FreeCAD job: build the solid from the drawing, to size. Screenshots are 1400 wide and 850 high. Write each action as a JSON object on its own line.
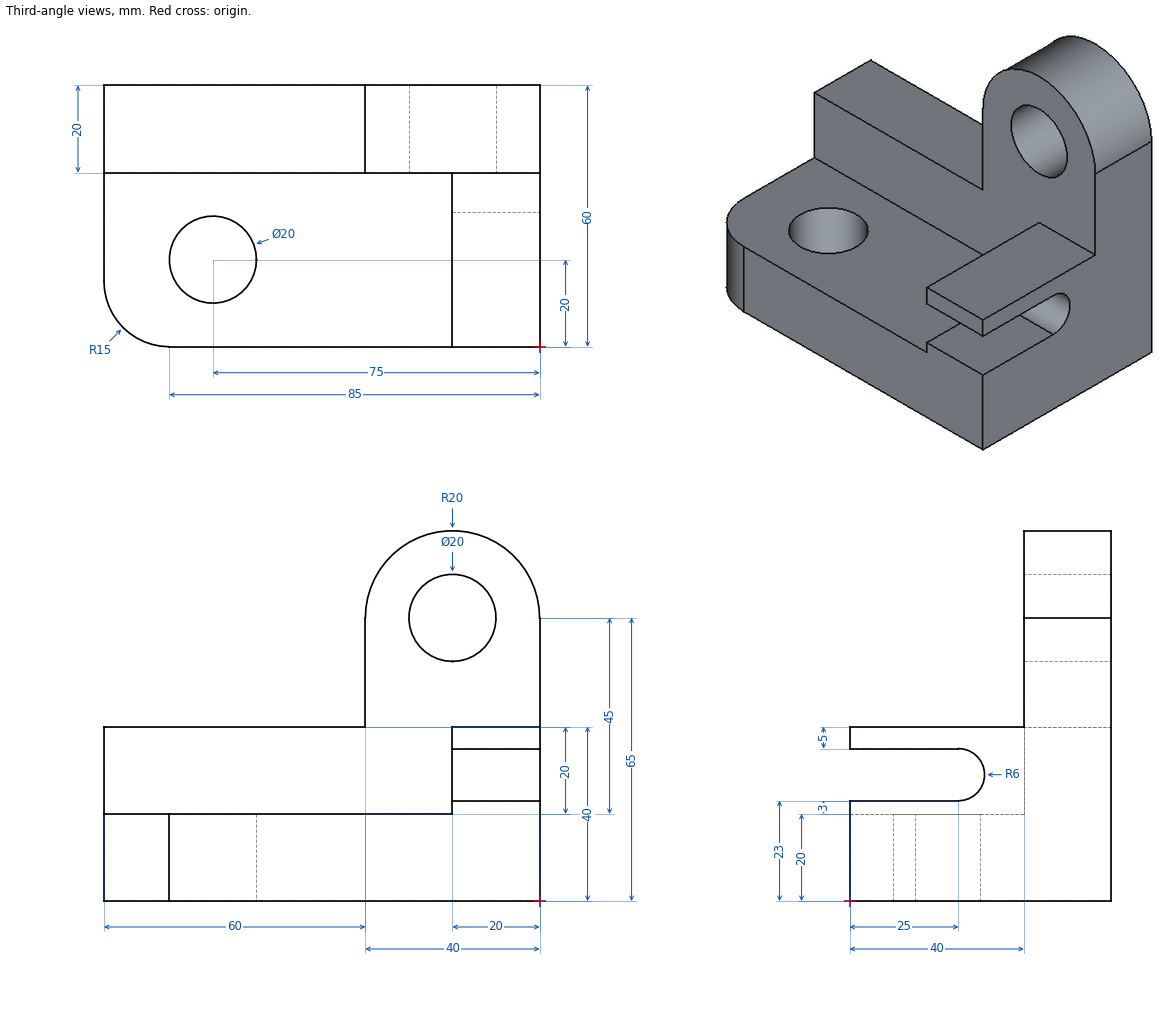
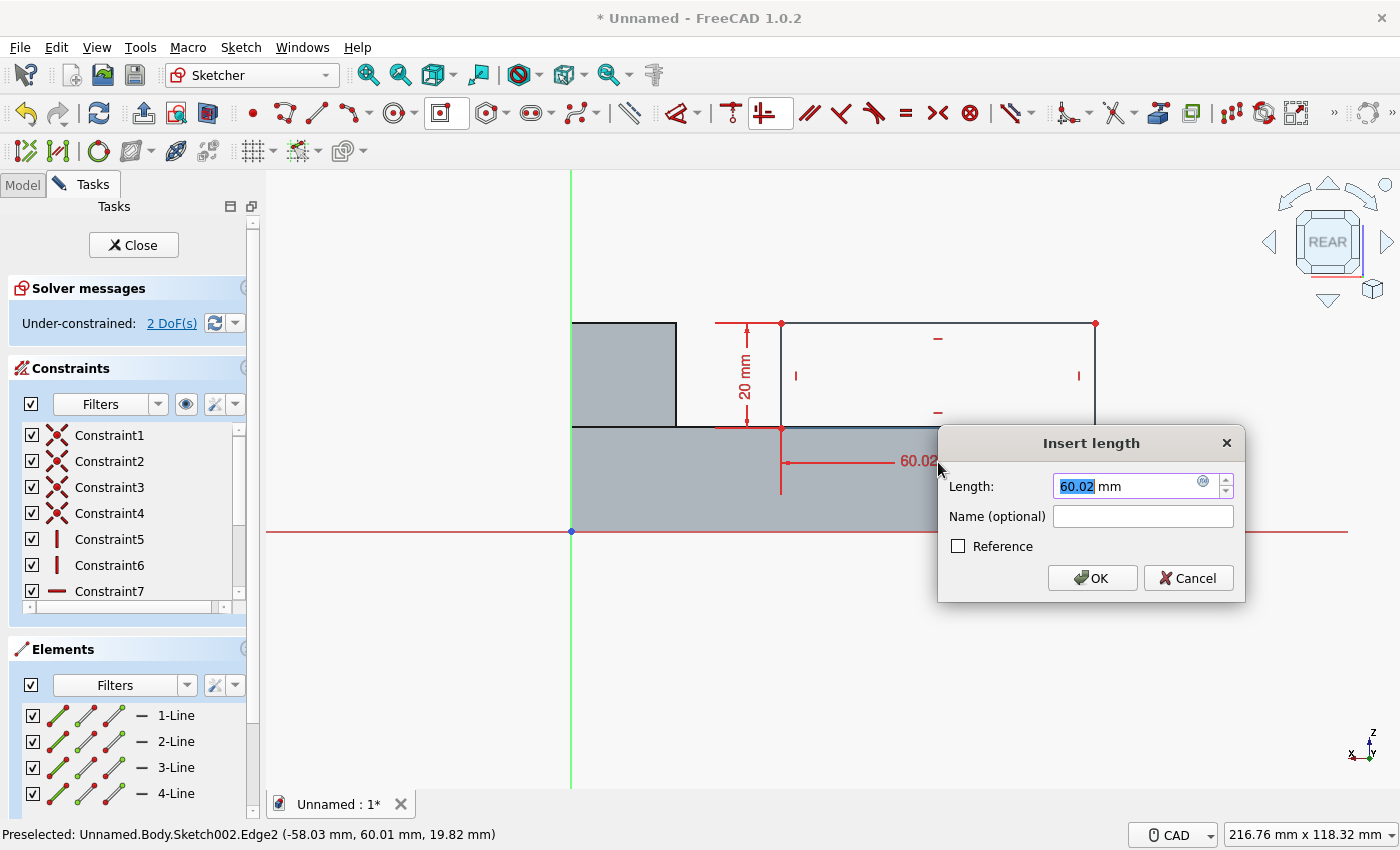
{"action": "type", "text": "60"}
{"action": "key", "text": "Return"}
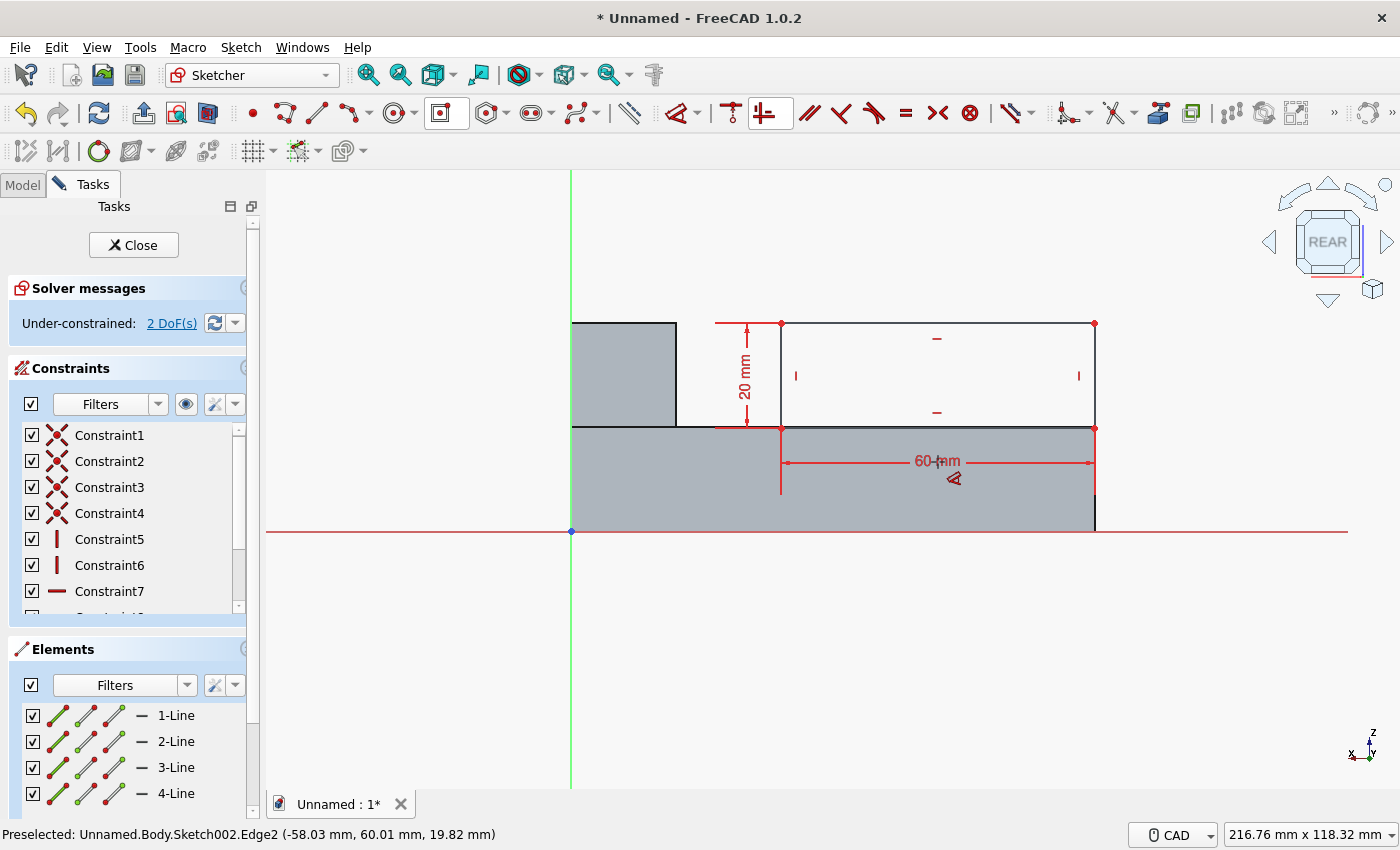
{"action": "left_click", "coordinate": [781, 323]}
{"action": "left_click", "coordinate": [676, 566]}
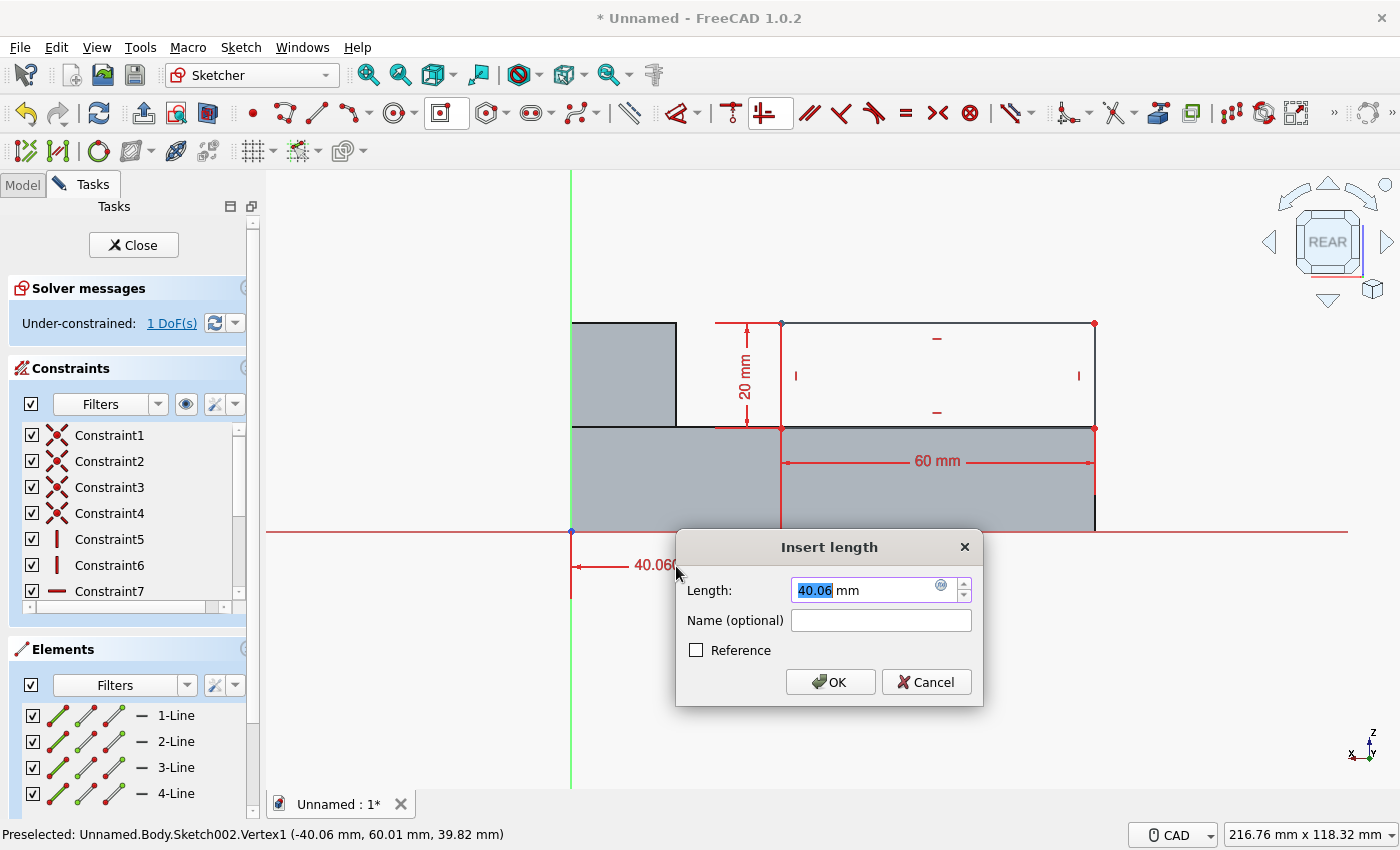
{"action": "type", "text": "40"}
{"action": "key", "text": "Return"}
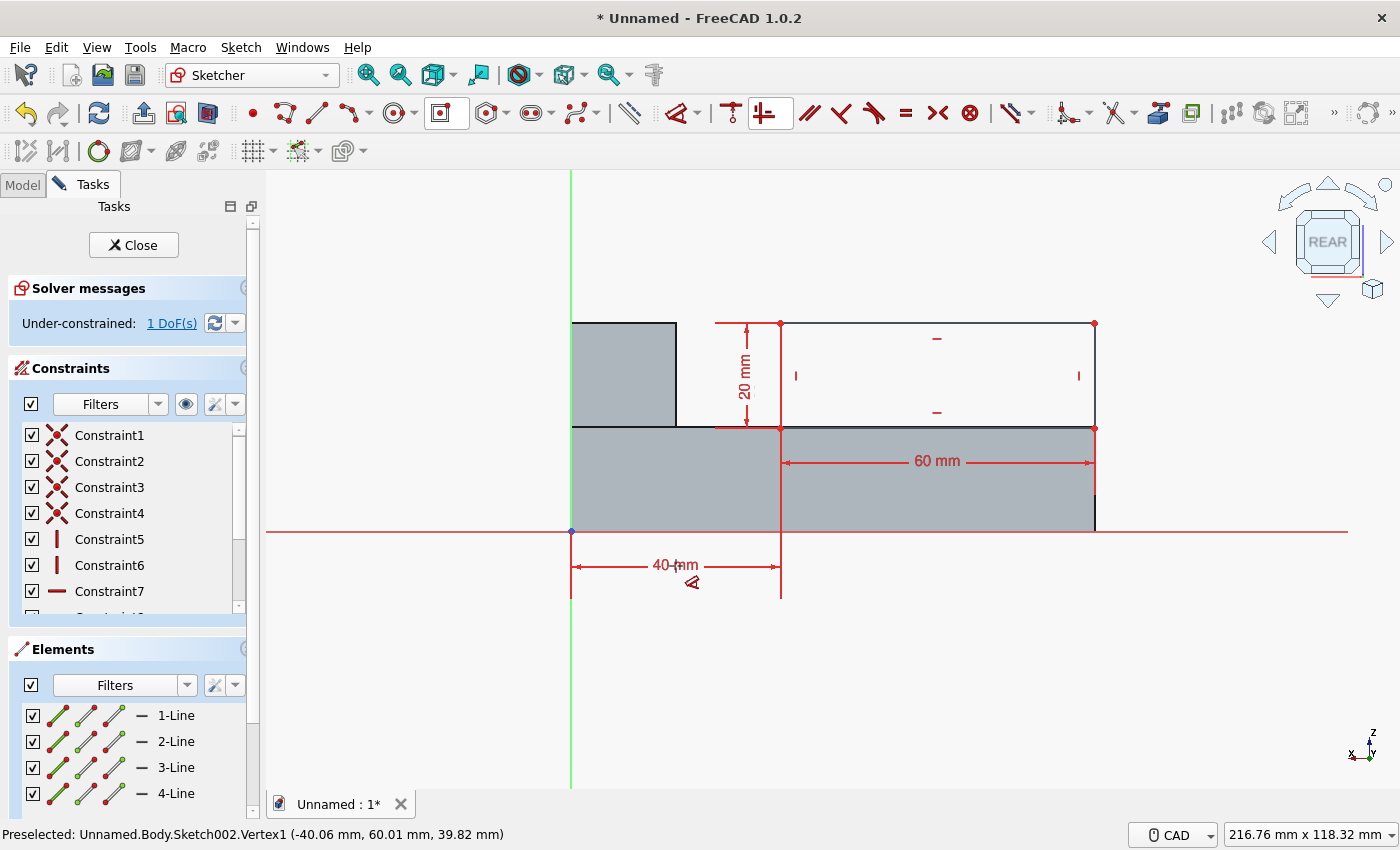
{"action": "left_click", "coordinate": [781, 323]}
{"action": "left_click", "coordinate": [537, 428]}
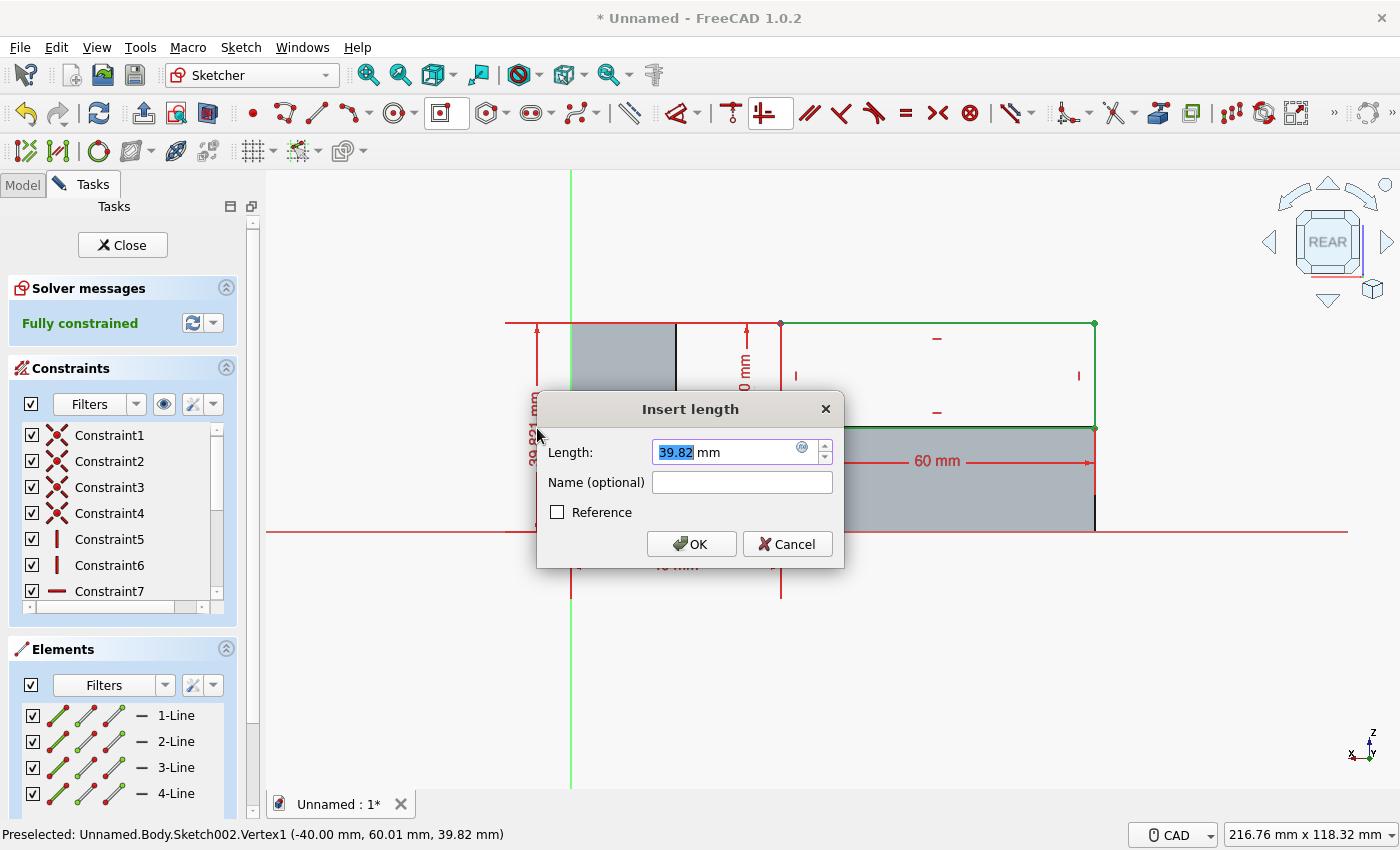
{"action": "type", "text": "40"}
{"action": "key", "text": "Return"}
{"action": "key", "text": "Escape"}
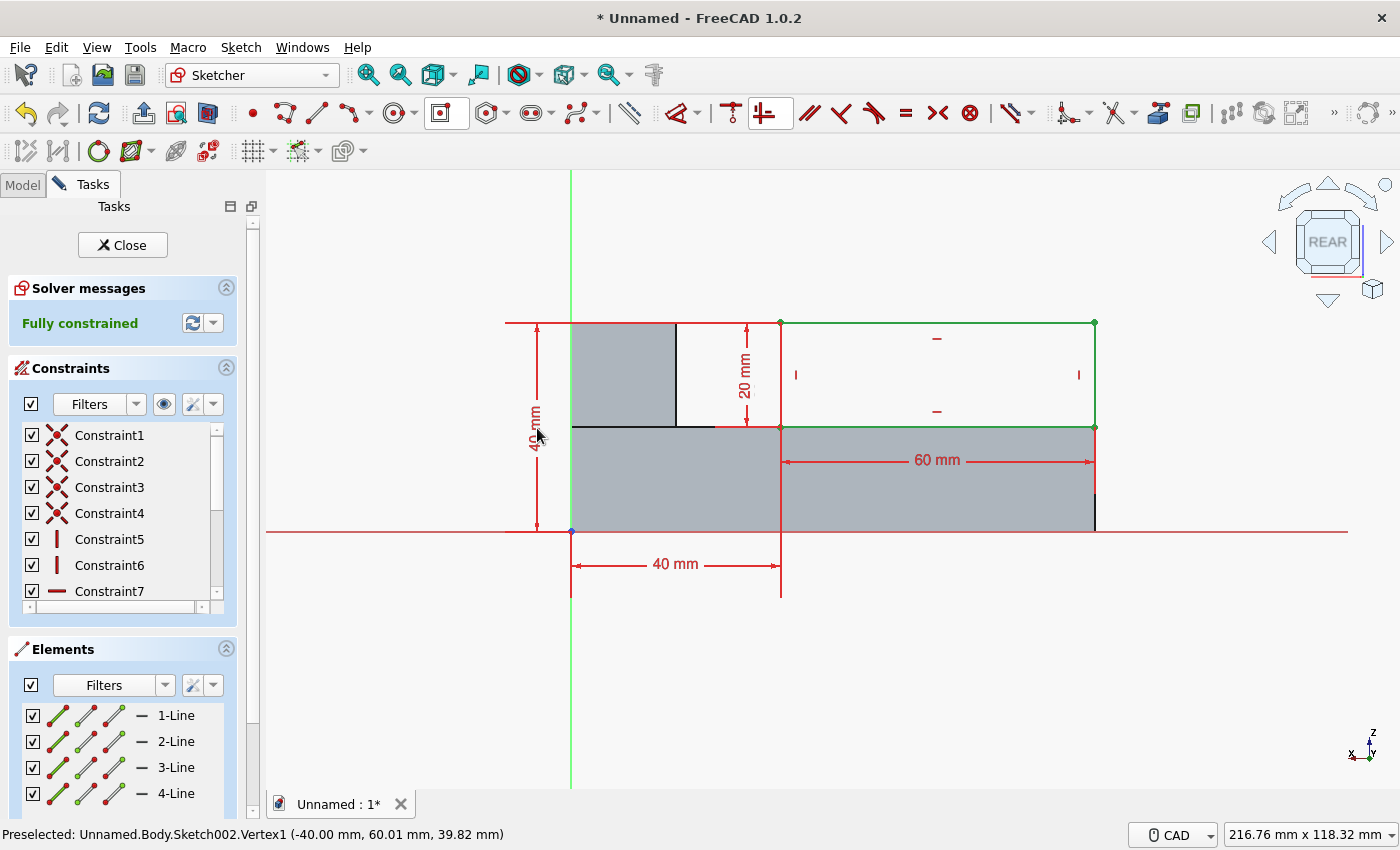
{"action": "left_click", "coordinate": [123, 245]}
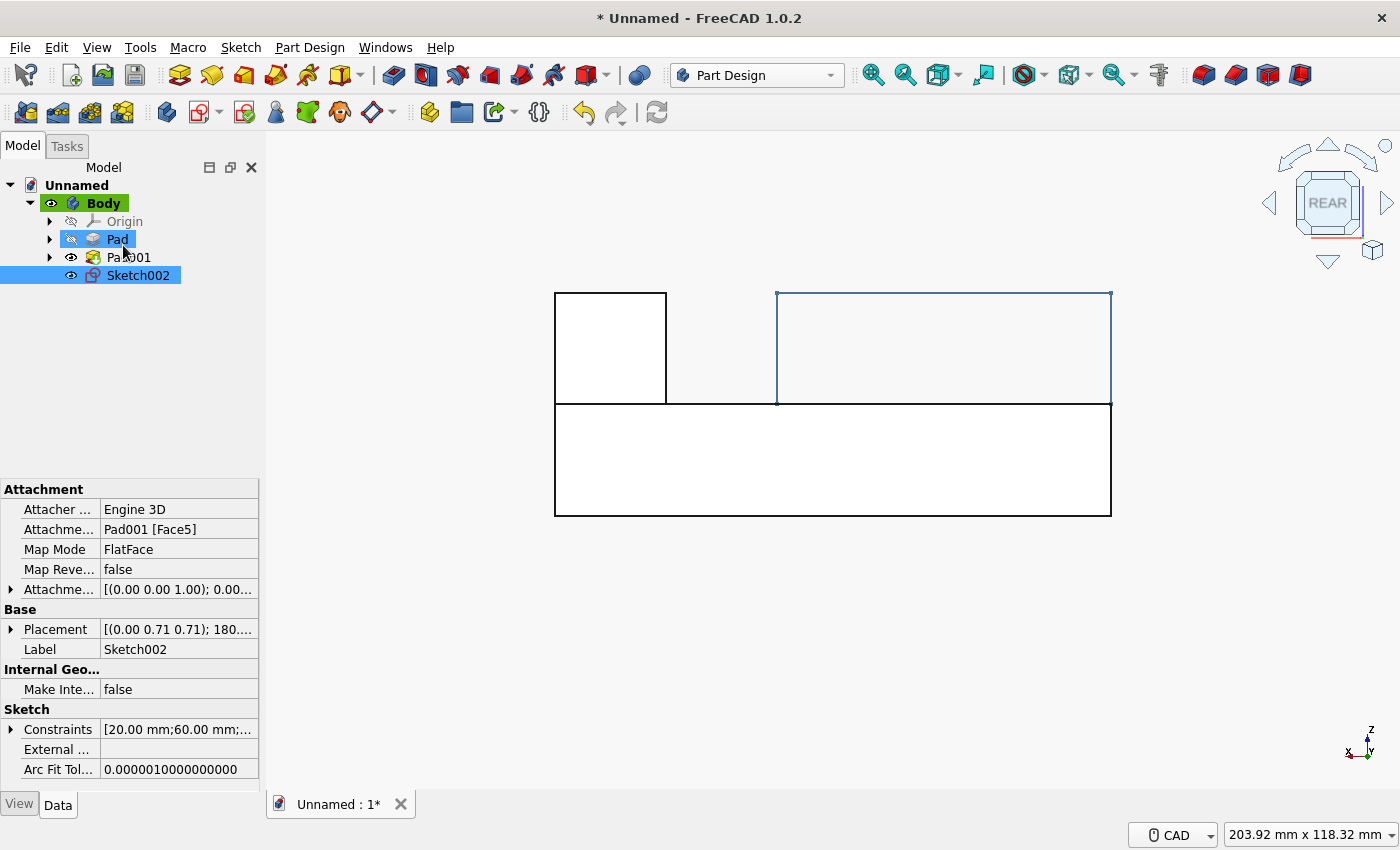
{"action": "left_click", "coordinate": [180, 76]}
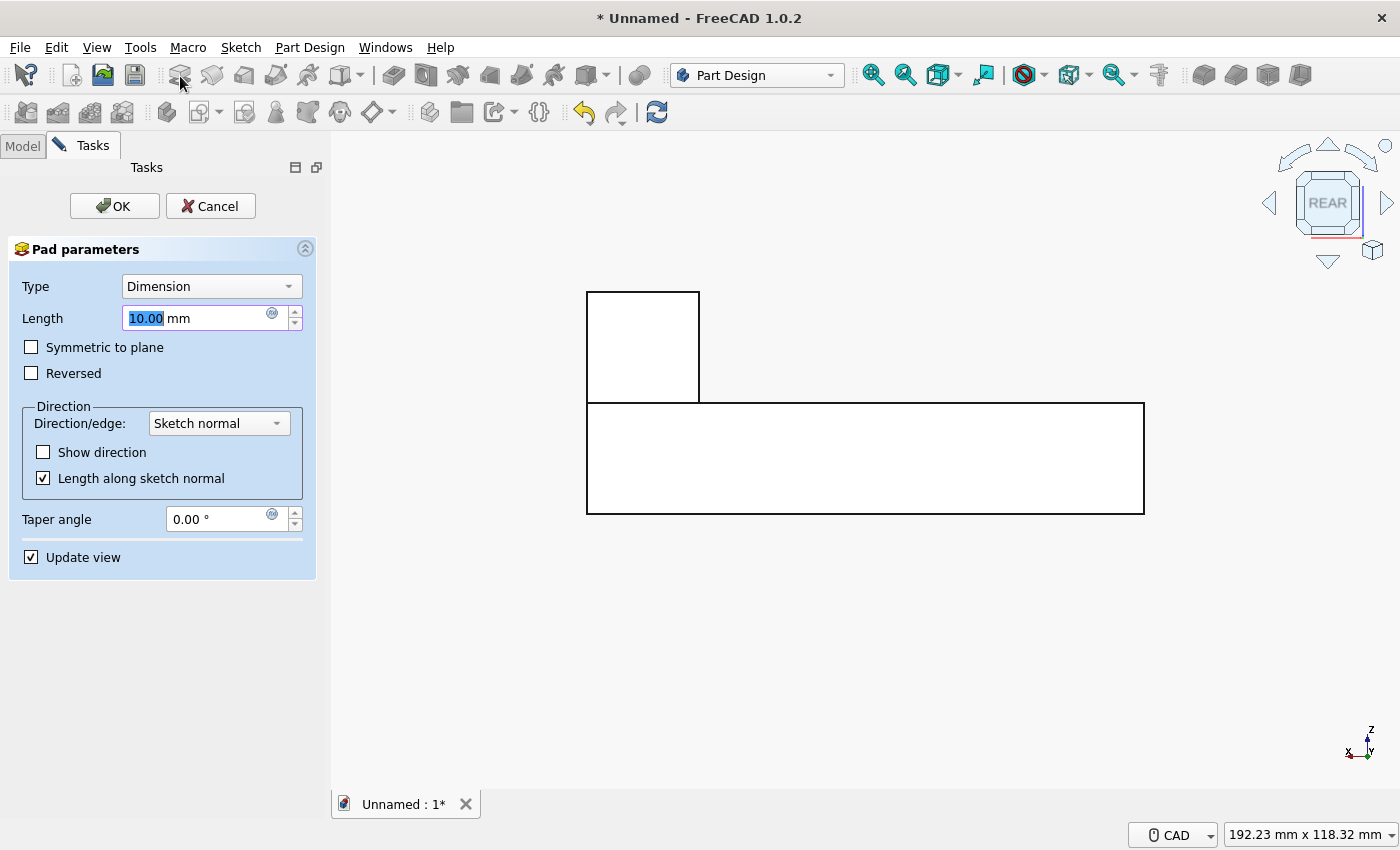
{"action": "type", "text": "20"}
{"action": "key", "text": "Tab"}